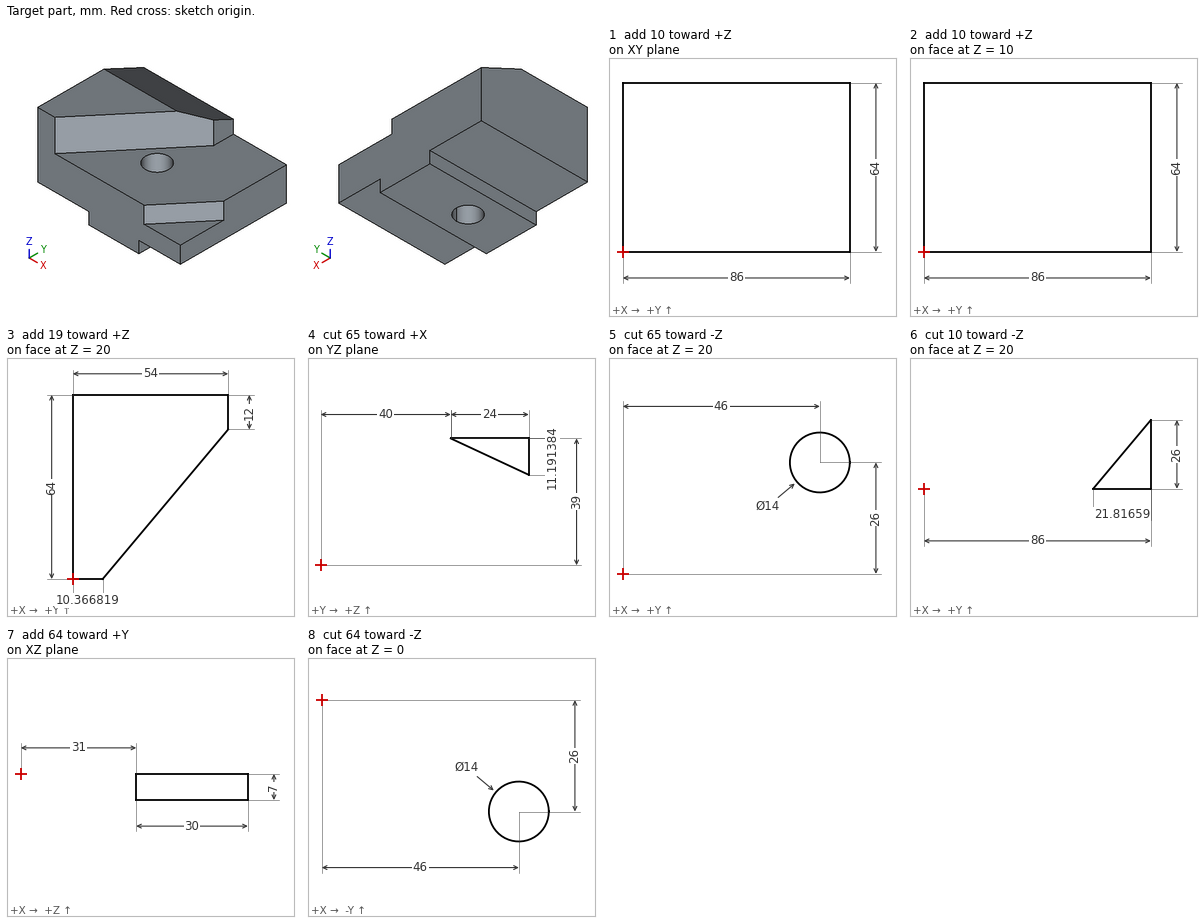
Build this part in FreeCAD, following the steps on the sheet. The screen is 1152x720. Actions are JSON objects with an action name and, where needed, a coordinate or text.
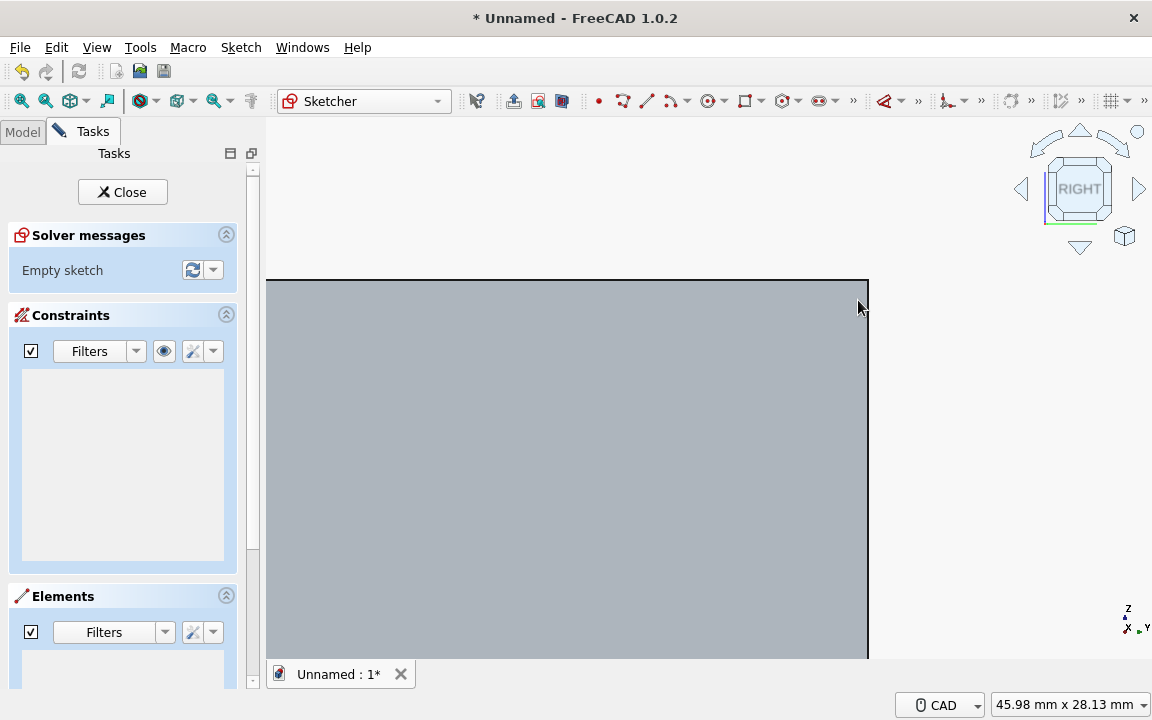
{"action": "left_click", "coordinate": [624, 102]}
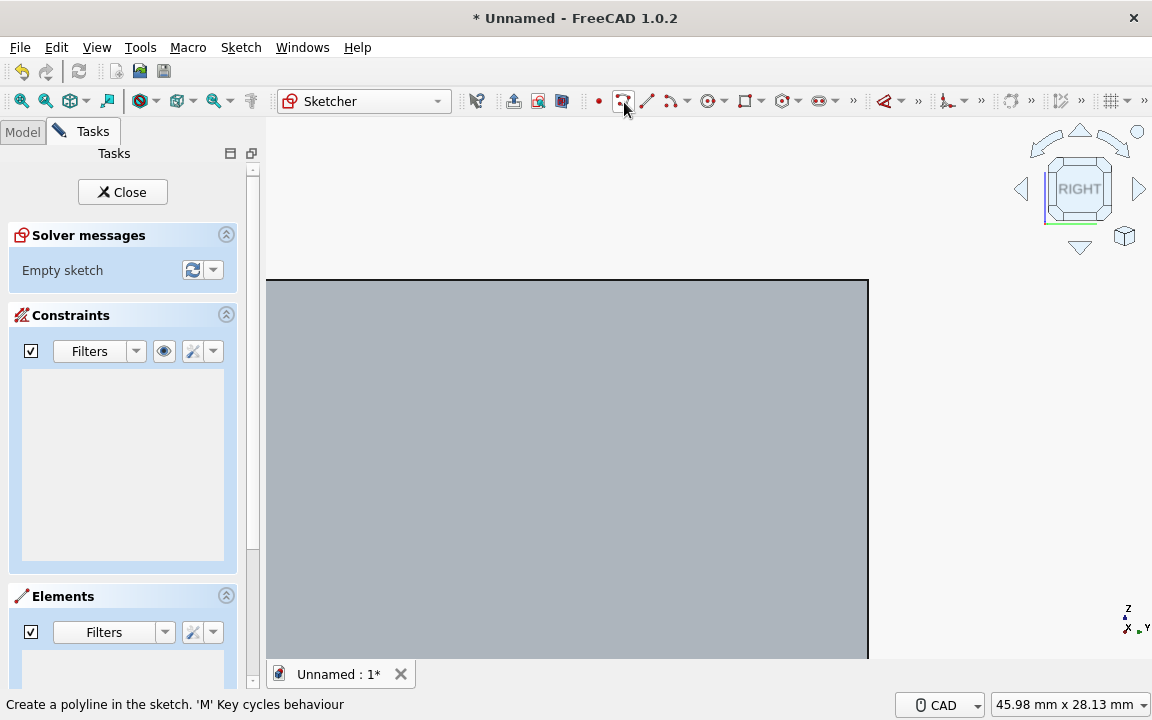
{"action": "left_click", "coordinate": [406, 280]}
{"action": "left_click", "coordinate": [868, 280]}
{"action": "left_click", "coordinate": [868, 496]}
{"action": "left_click", "coordinate": [406, 281]}
{"action": "key", "text": "Escape"}
{"action": "key", "text": "Escape"}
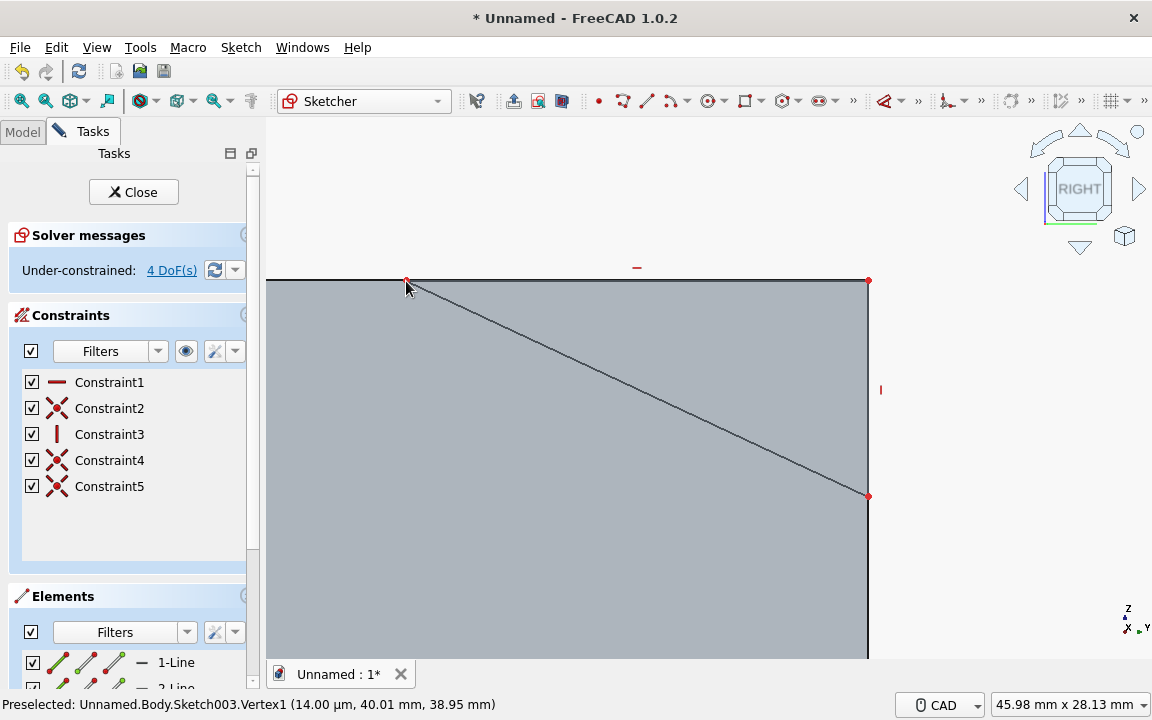
{"action": "left_click", "coordinate": [884, 102]}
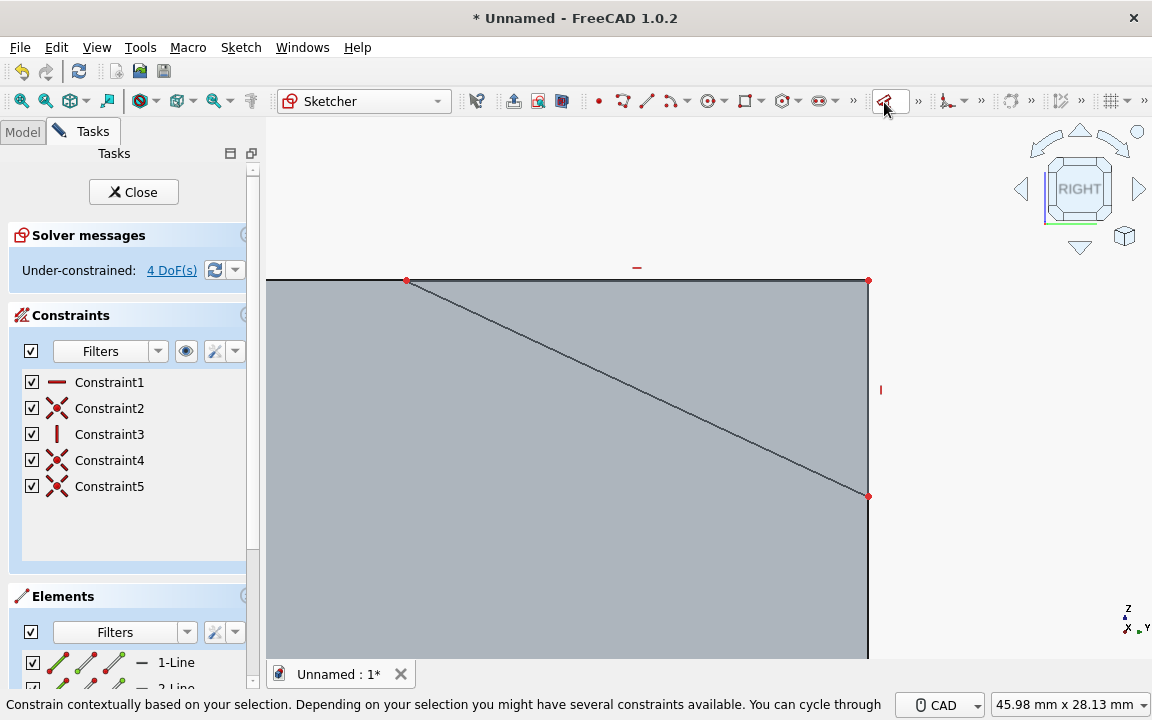
{"action": "left_click", "coordinate": [545, 281]}
{"action": "left_click", "coordinate": [637, 247]}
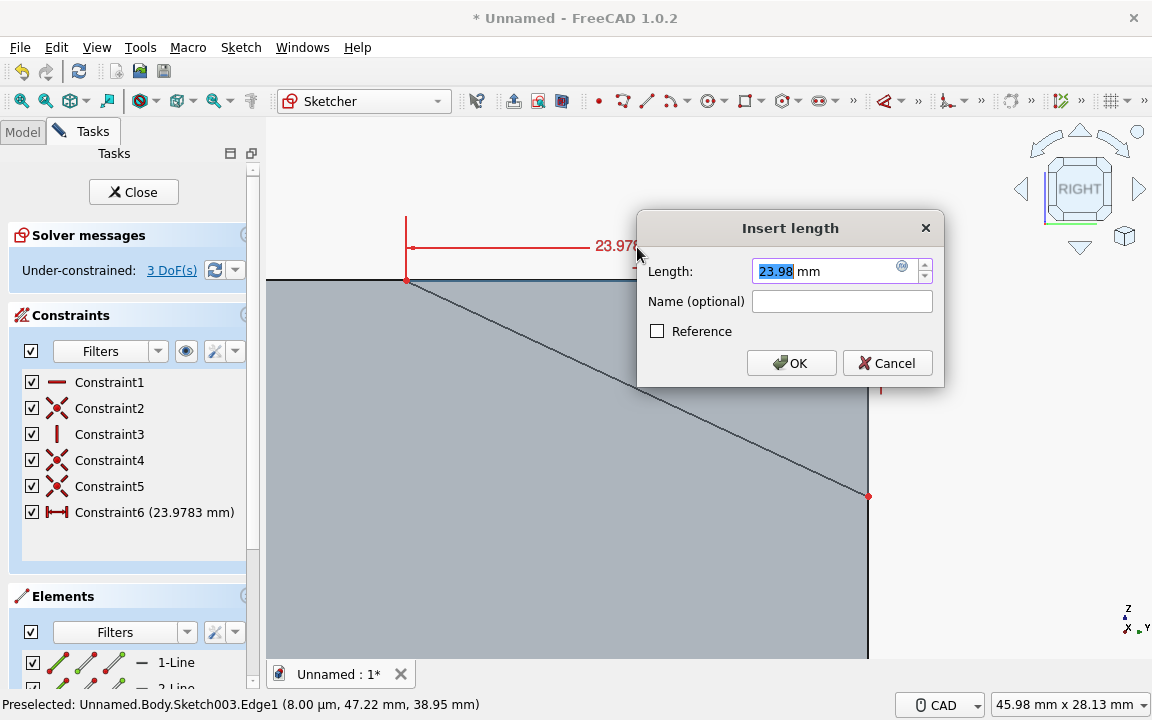
{"action": "type", "text": "24"}
{"action": "key", "text": "Return"}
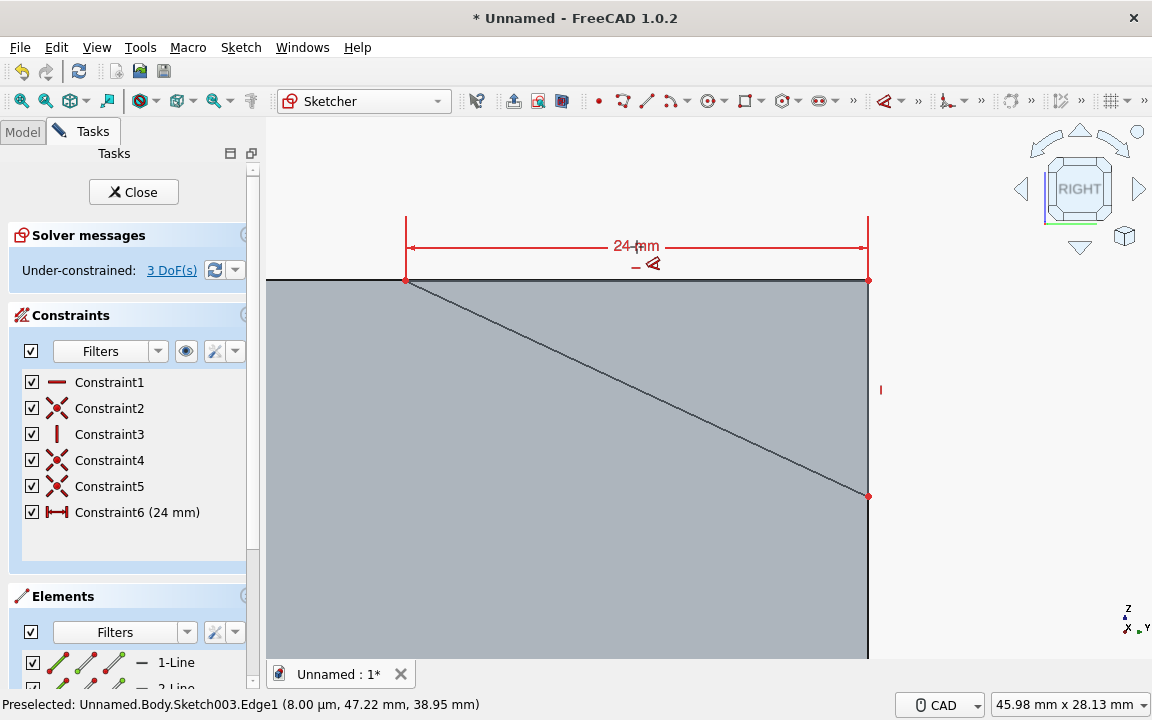
{"action": "left_click", "coordinate": [406, 281]}
{"action": "left_click", "coordinate": [350, 247]}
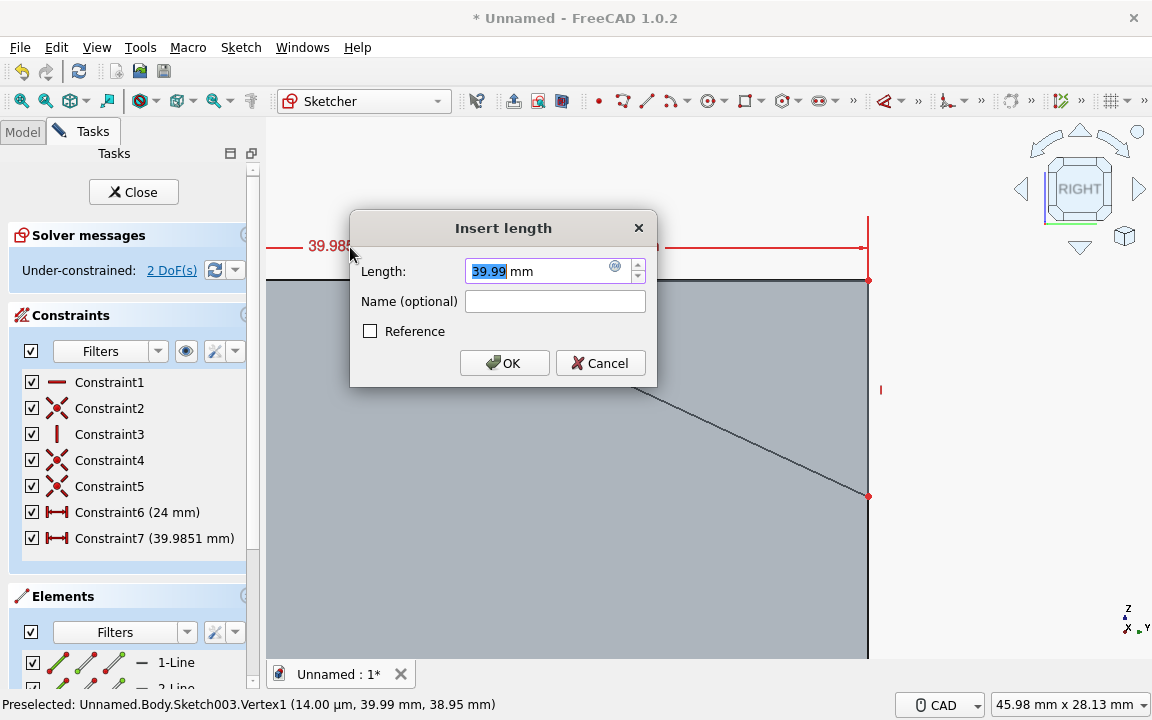
{"action": "type", "text": "40"}
{"action": "key", "text": "Return"}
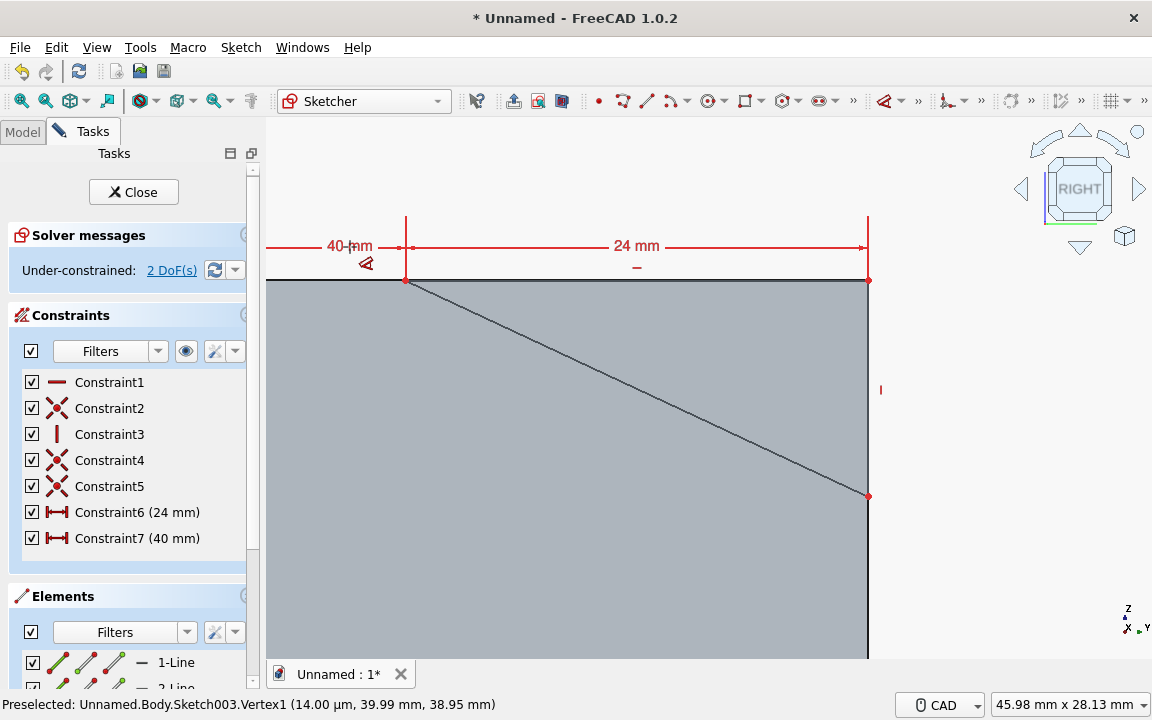
{"action": "left_click", "coordinate": [406, 281]}
{"action": "left_click", "coordinate": [440, 456]}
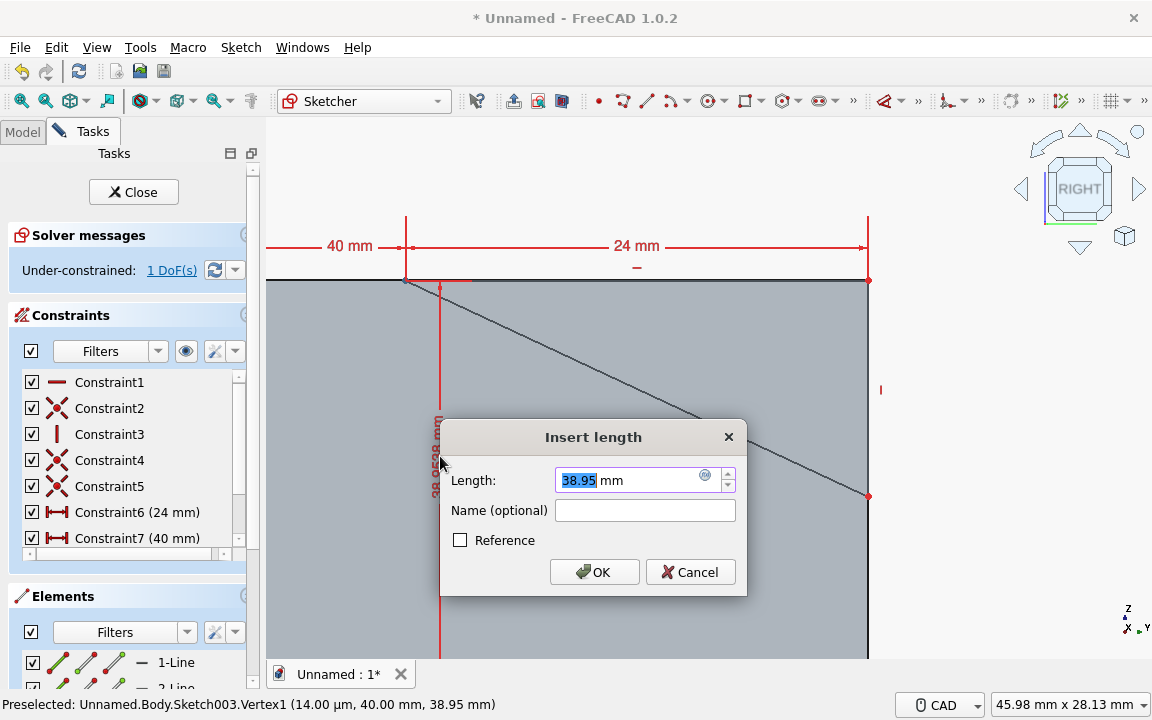
{"action": "type", "text": "39"}
{"action": "key", "text": "Return"}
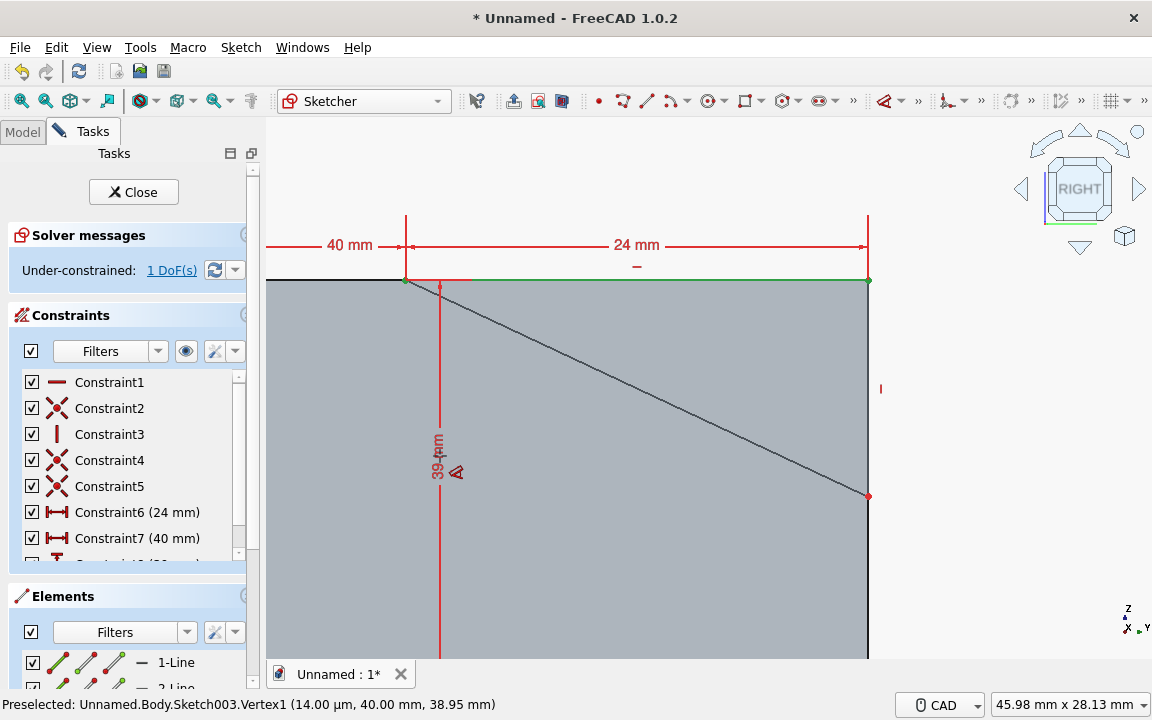
{"action": "left_click", "coordinate": [868, 345]}
{"action": "left_click", "coordinate": [902, 389]}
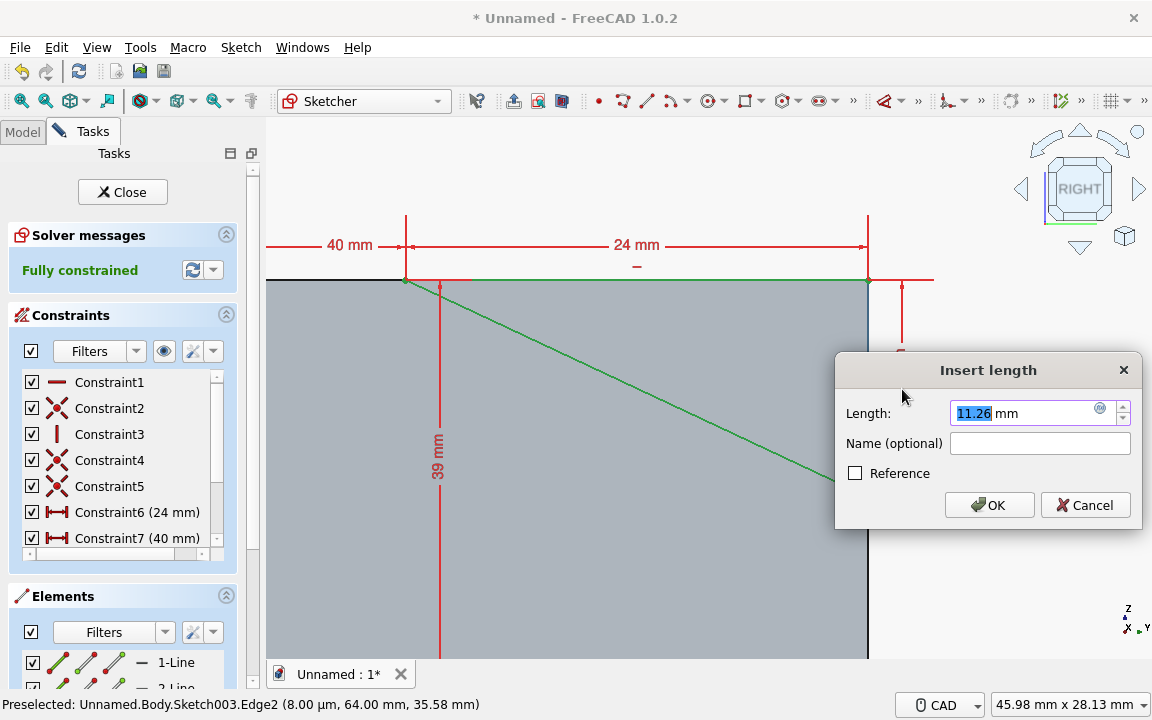
{"action": "type", "text": "11.191384"}
{"action": "key", "text": "Return"}
{"action": "key", "text": "Escape"}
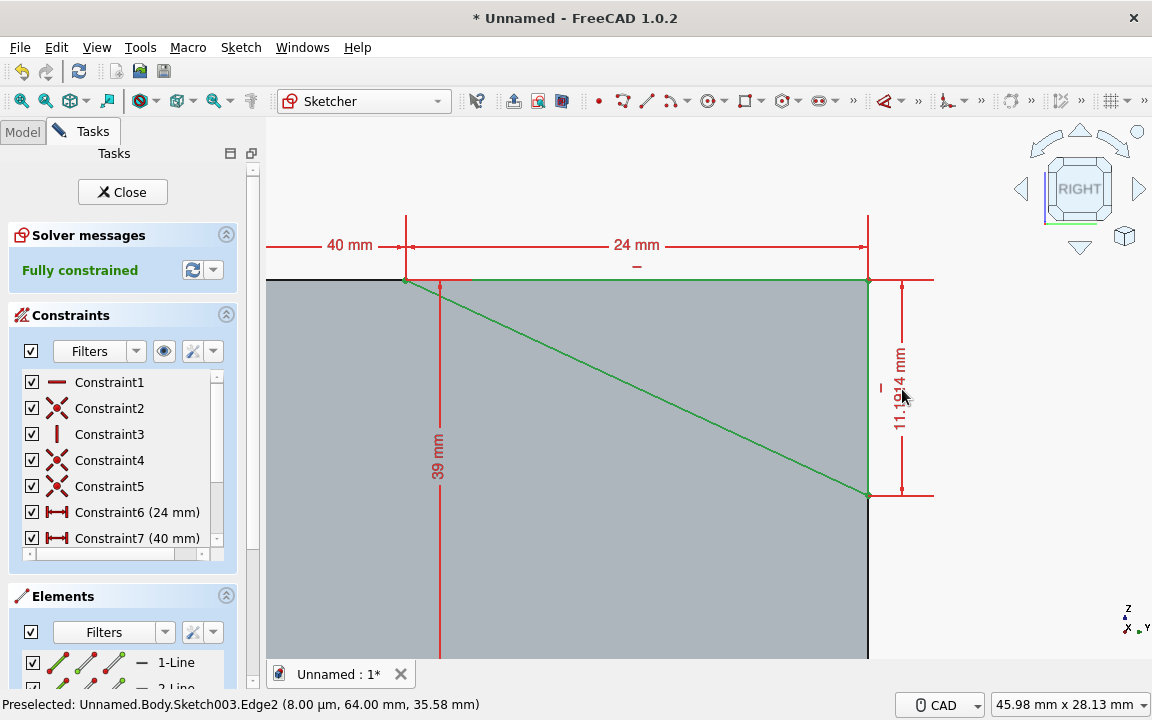
{"action": "left_click", "coordinate": [123, 192]}